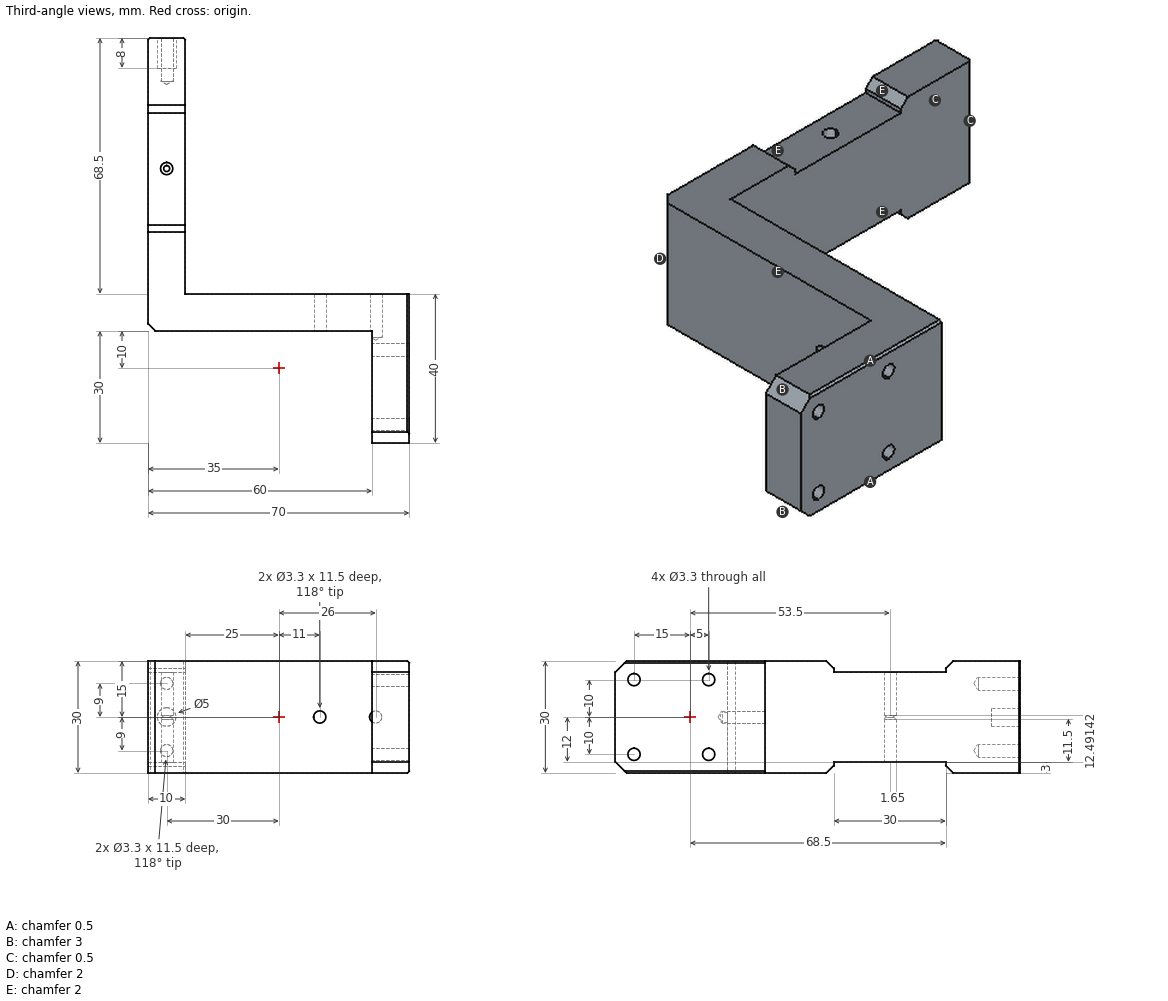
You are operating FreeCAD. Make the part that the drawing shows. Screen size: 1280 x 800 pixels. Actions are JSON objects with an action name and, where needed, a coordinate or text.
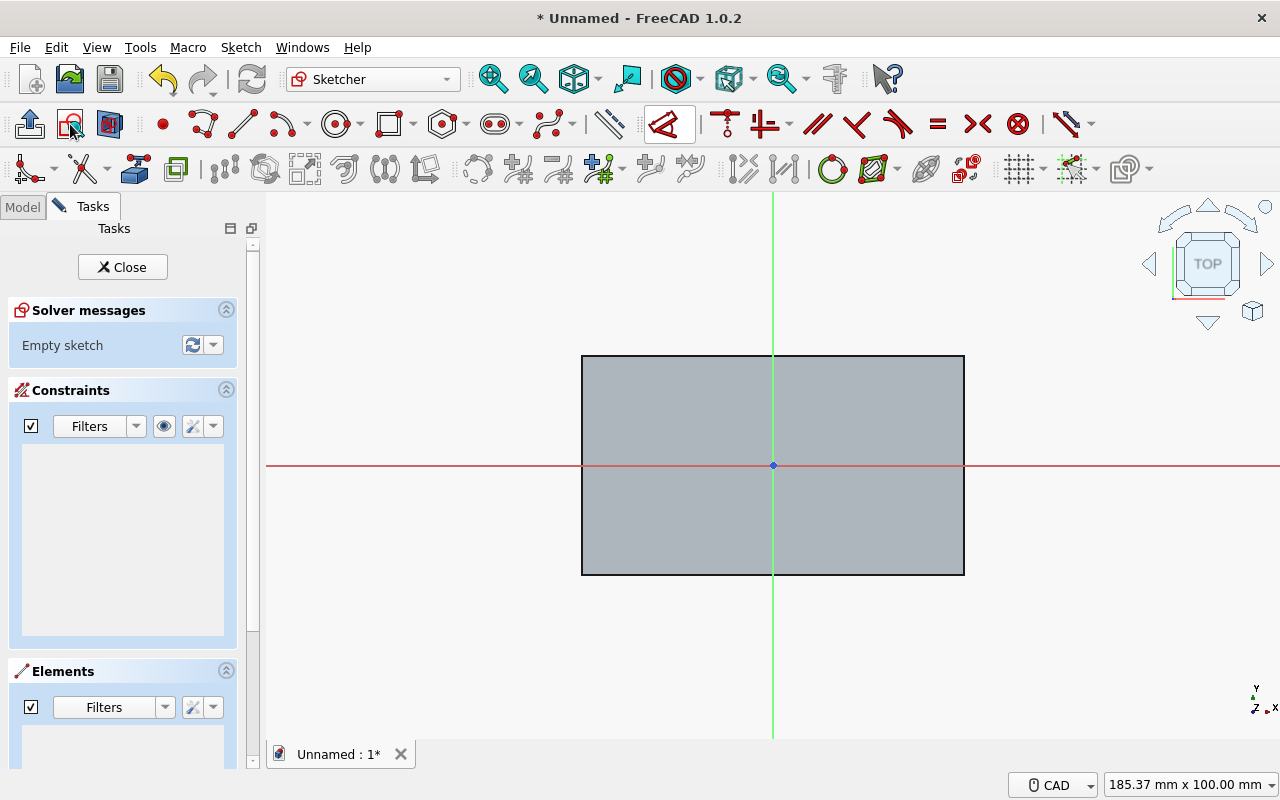
{"action": "scroll", "coordinate": [796, 526], "scroll_direction": "up", "scroll_amount": 3}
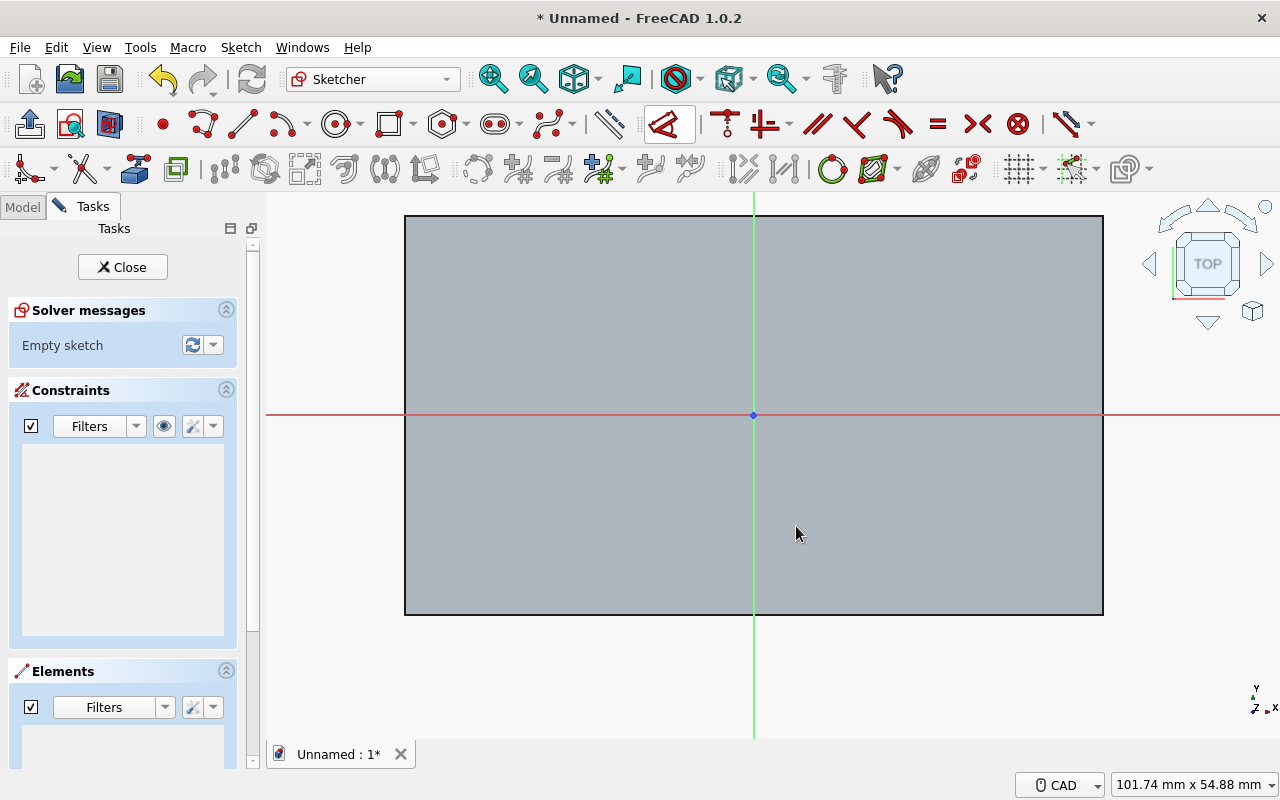
{"action": "left_click", "coordinate": [390, 124]}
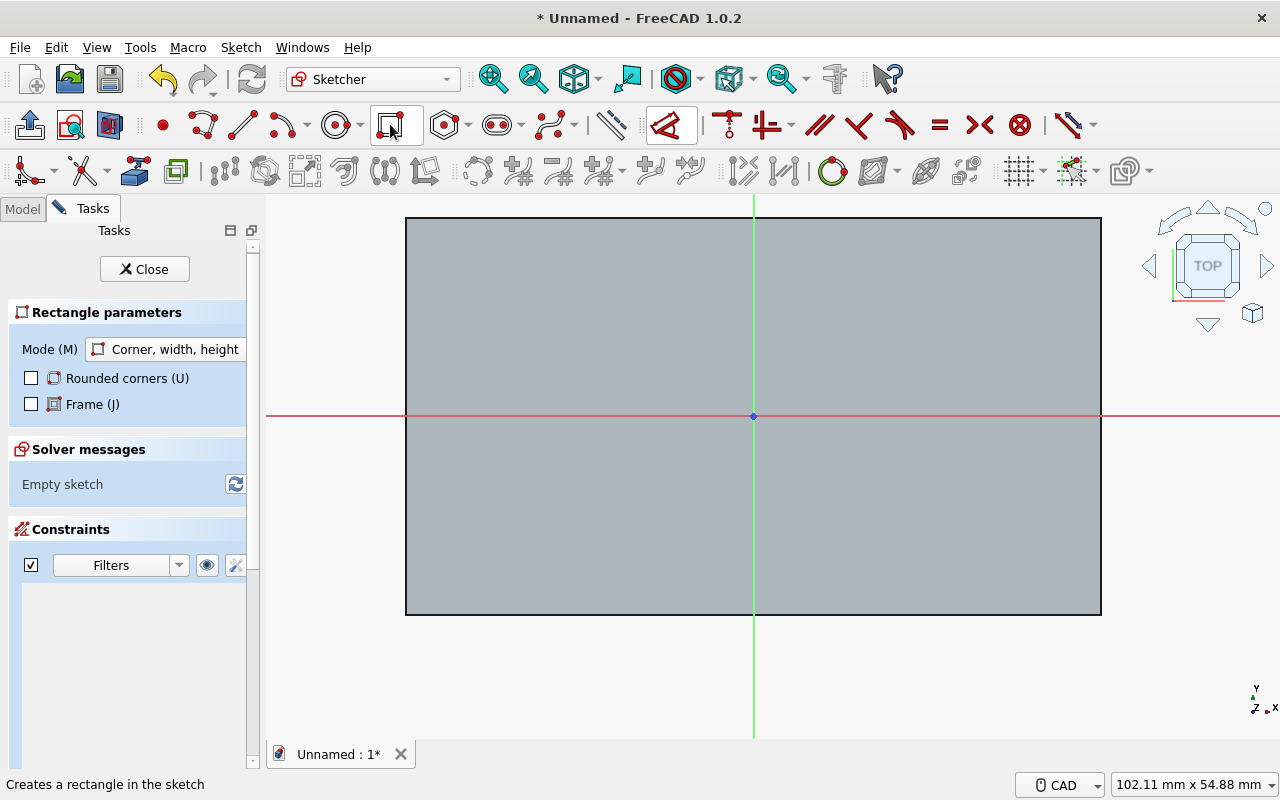
{"action": "left_click", "coordinate": [406, 317]}
{"action": "left_click", "coordinate": [1002, 615]}
{"action": "key", "text": "Escape"}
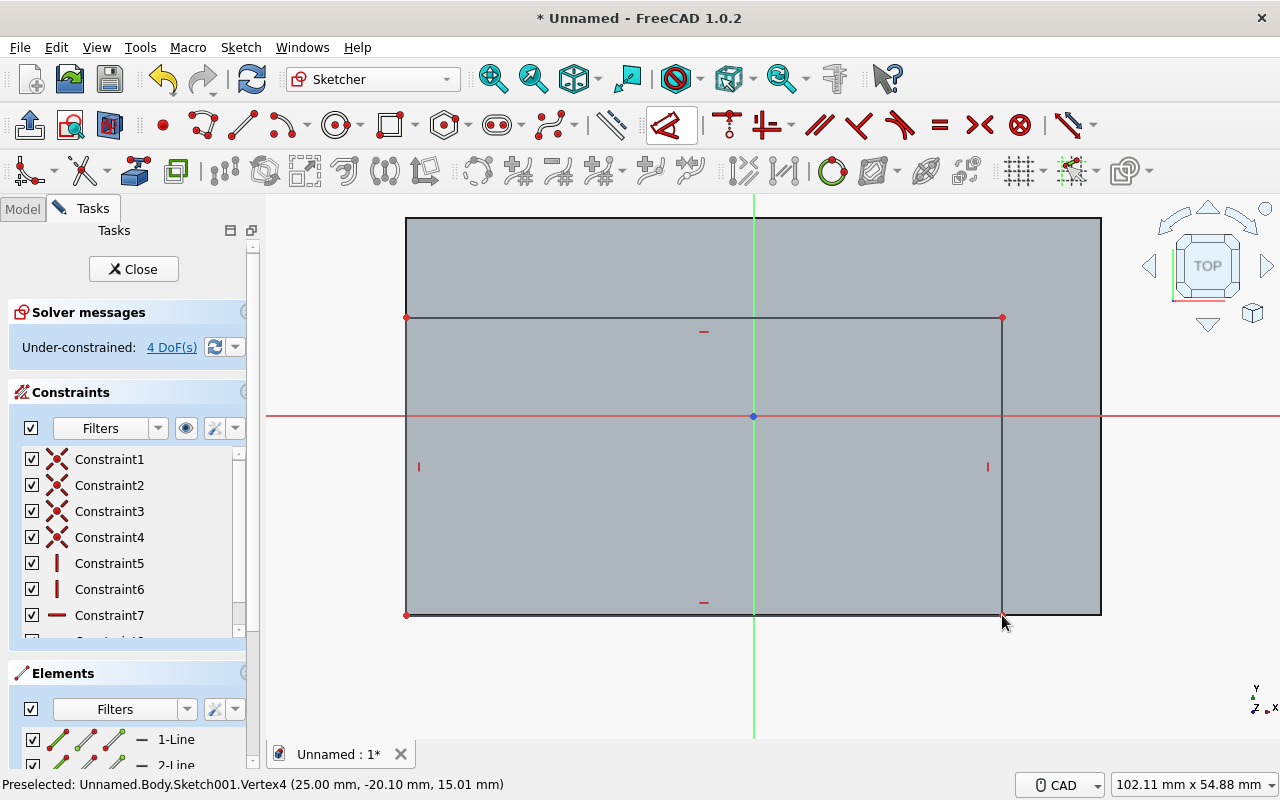
{"action": "scroll", "coordinate": [406, 407], "scroll_direction": "up", "scroll_amount": 3}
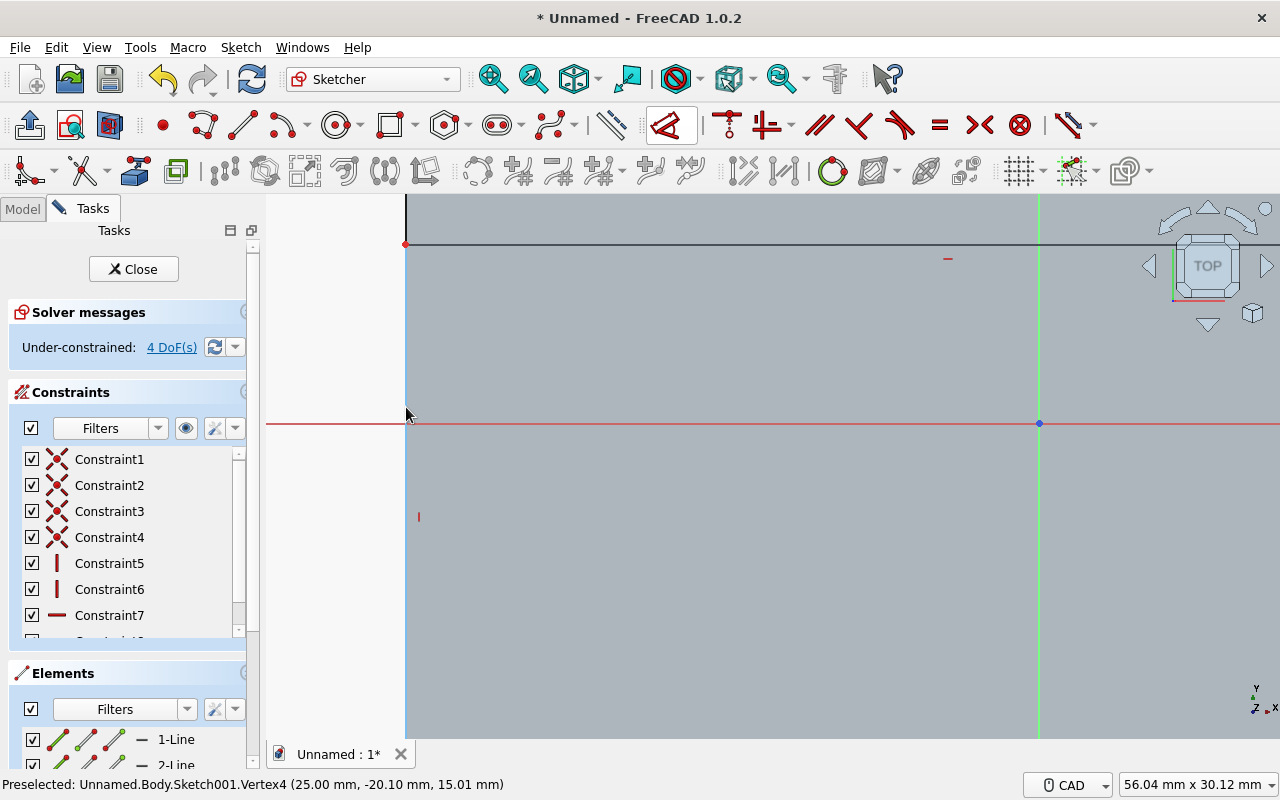
{"action": "left_click", "coordinate": [406, 407]}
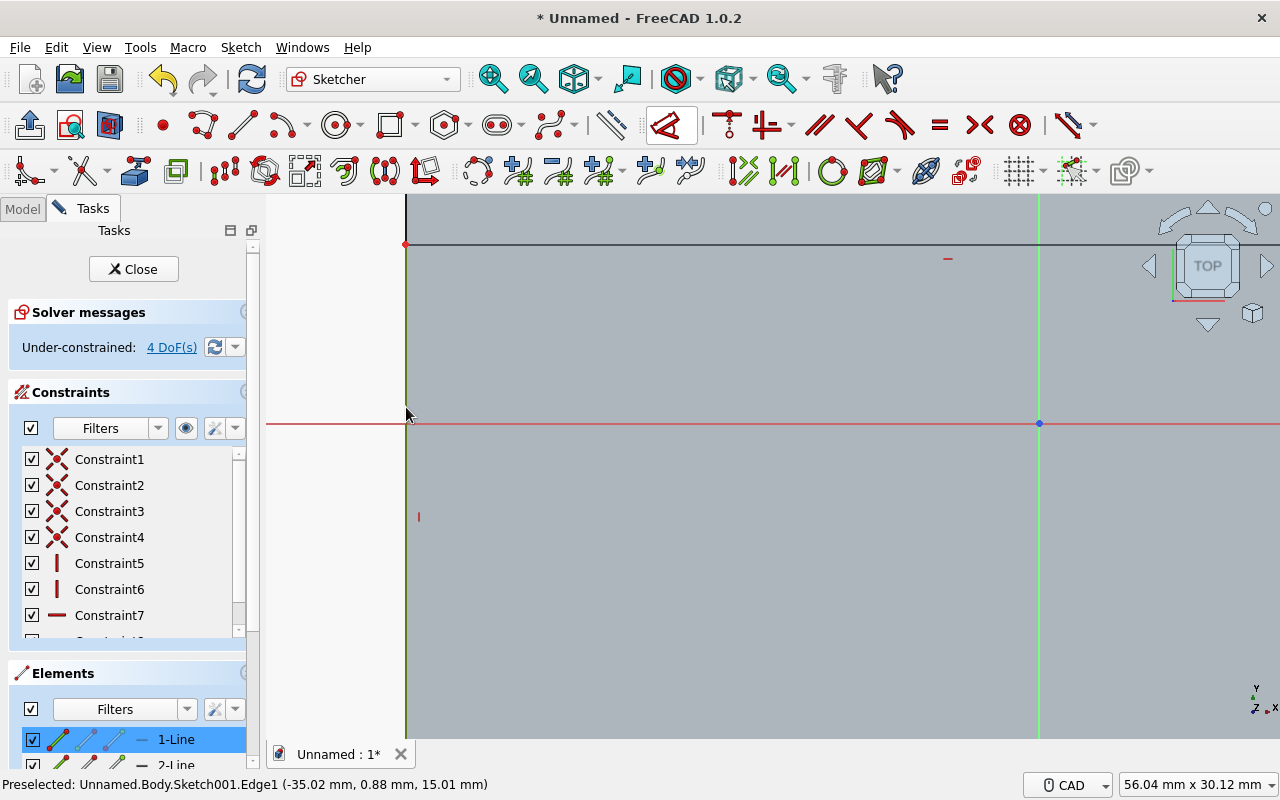
{"action": "left_click", "coordinate": [692, 126]}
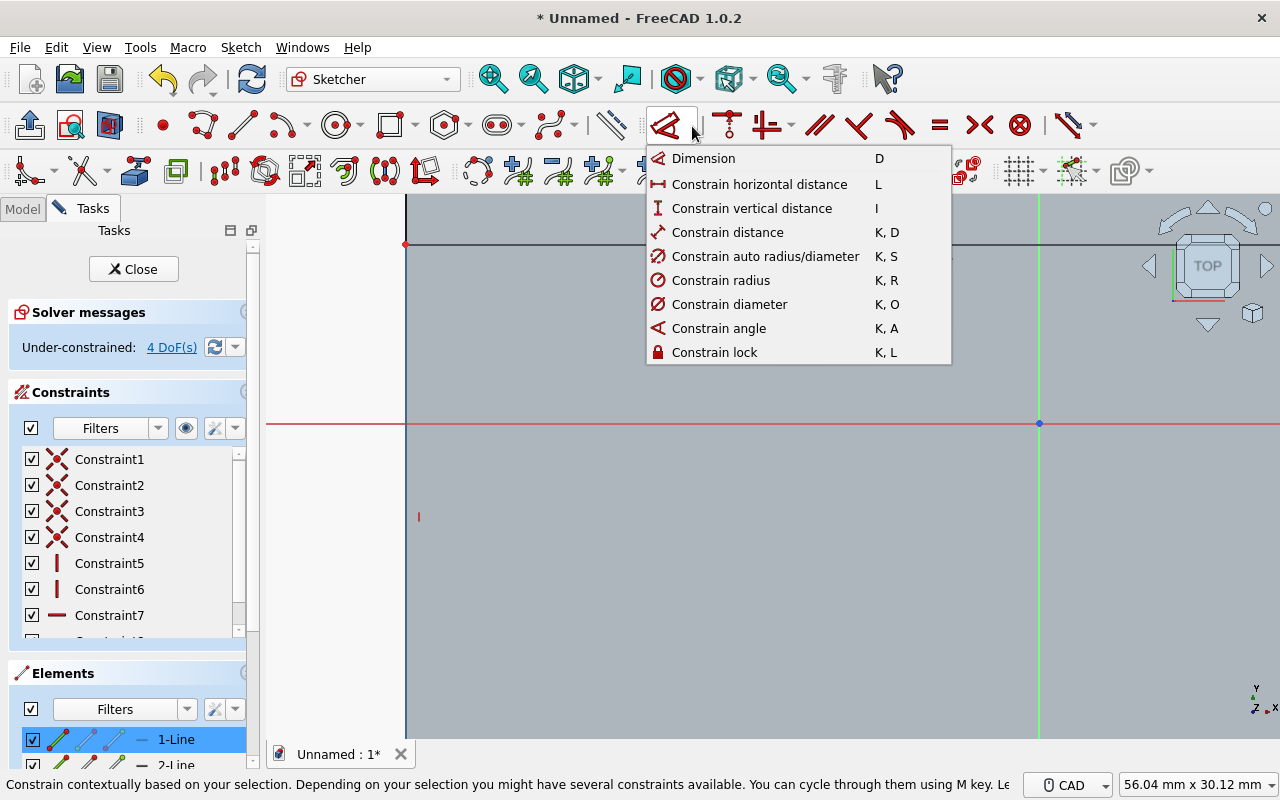
{"action": "left_click", "coordinate": [799, 208]}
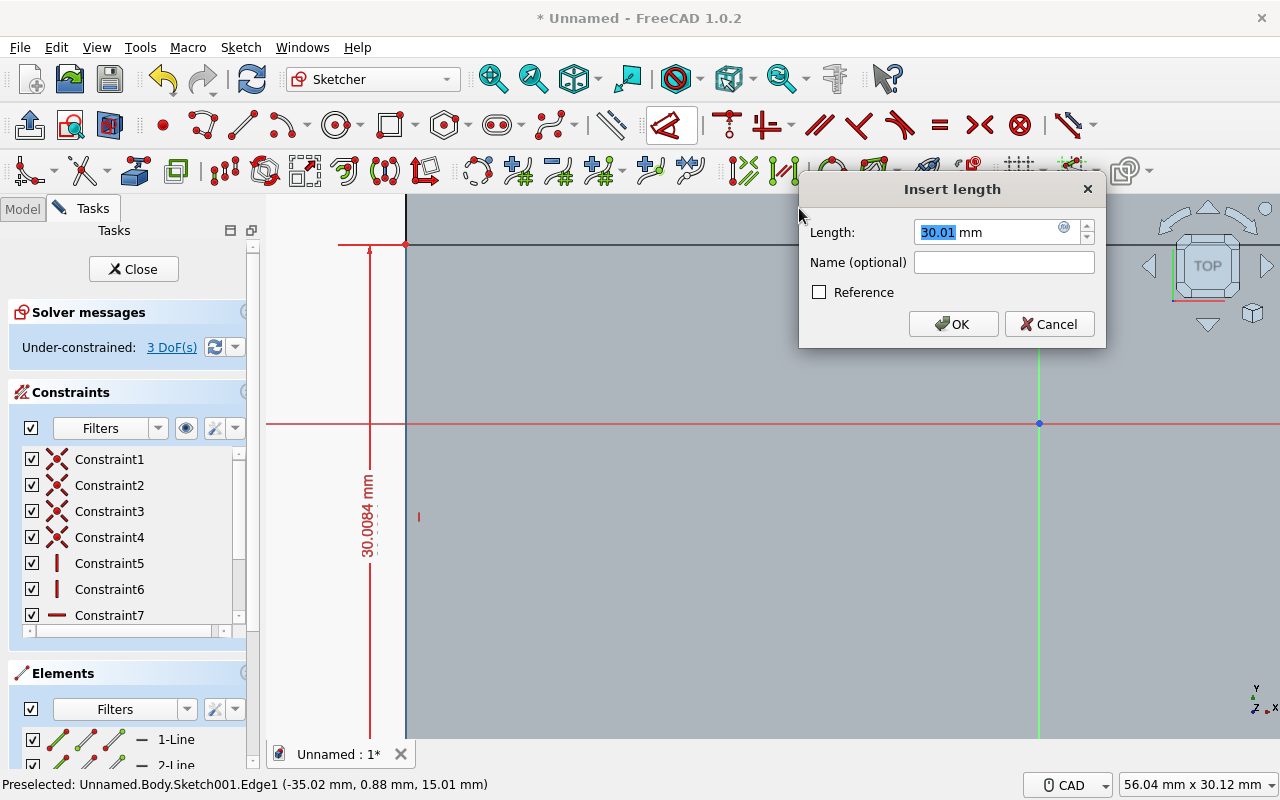
{"action": "type", "text": "30"}
{"action": "key", "text": "Return"}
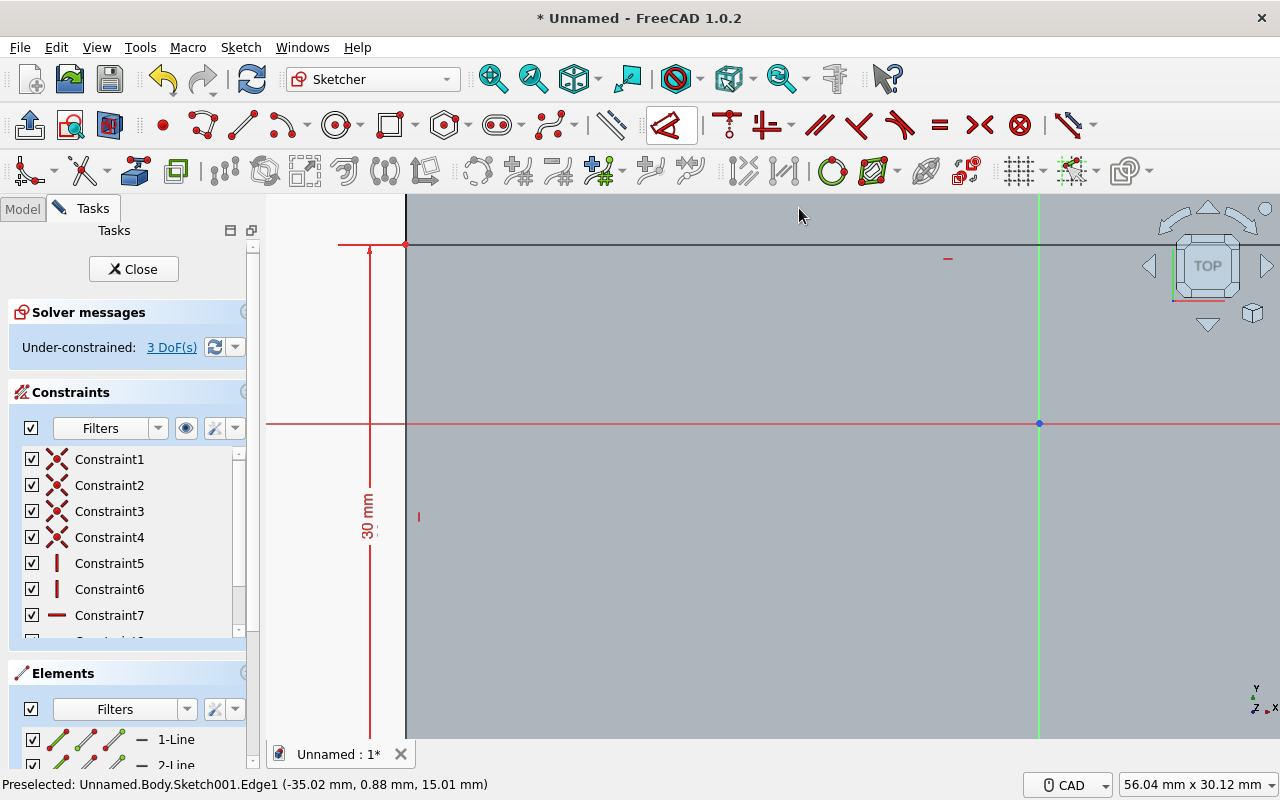
{"action": "scroll", "coordinate": [407, 408], "scroll_direction": "down", "scroll_amount": 3}